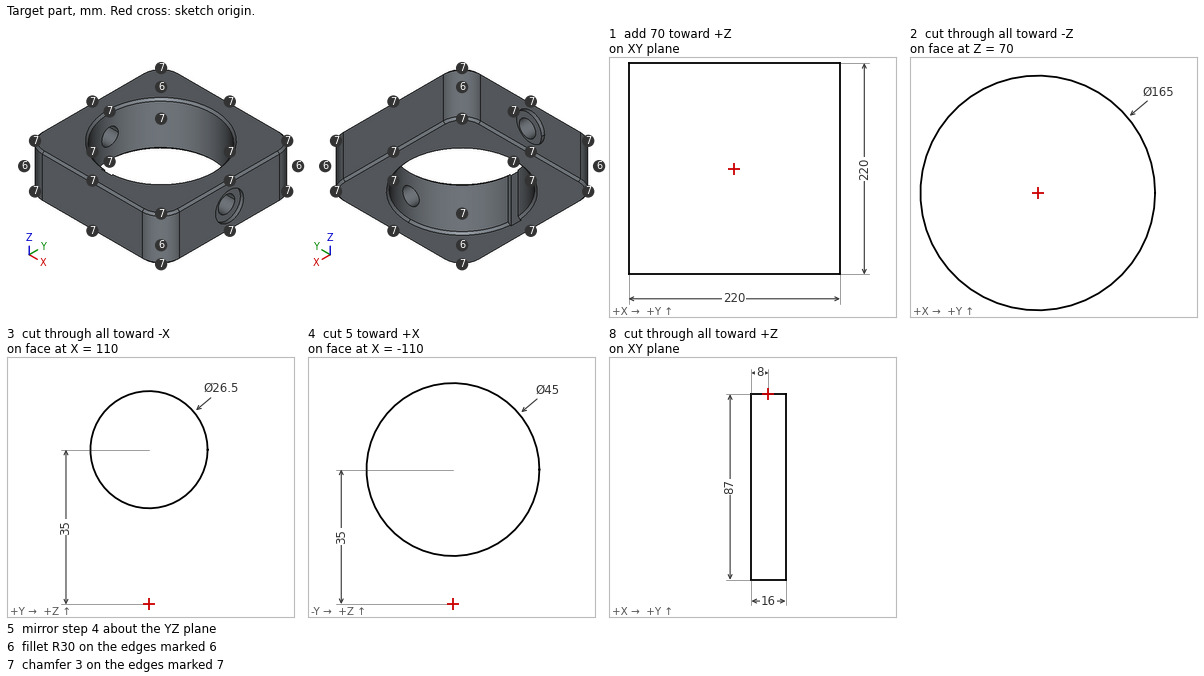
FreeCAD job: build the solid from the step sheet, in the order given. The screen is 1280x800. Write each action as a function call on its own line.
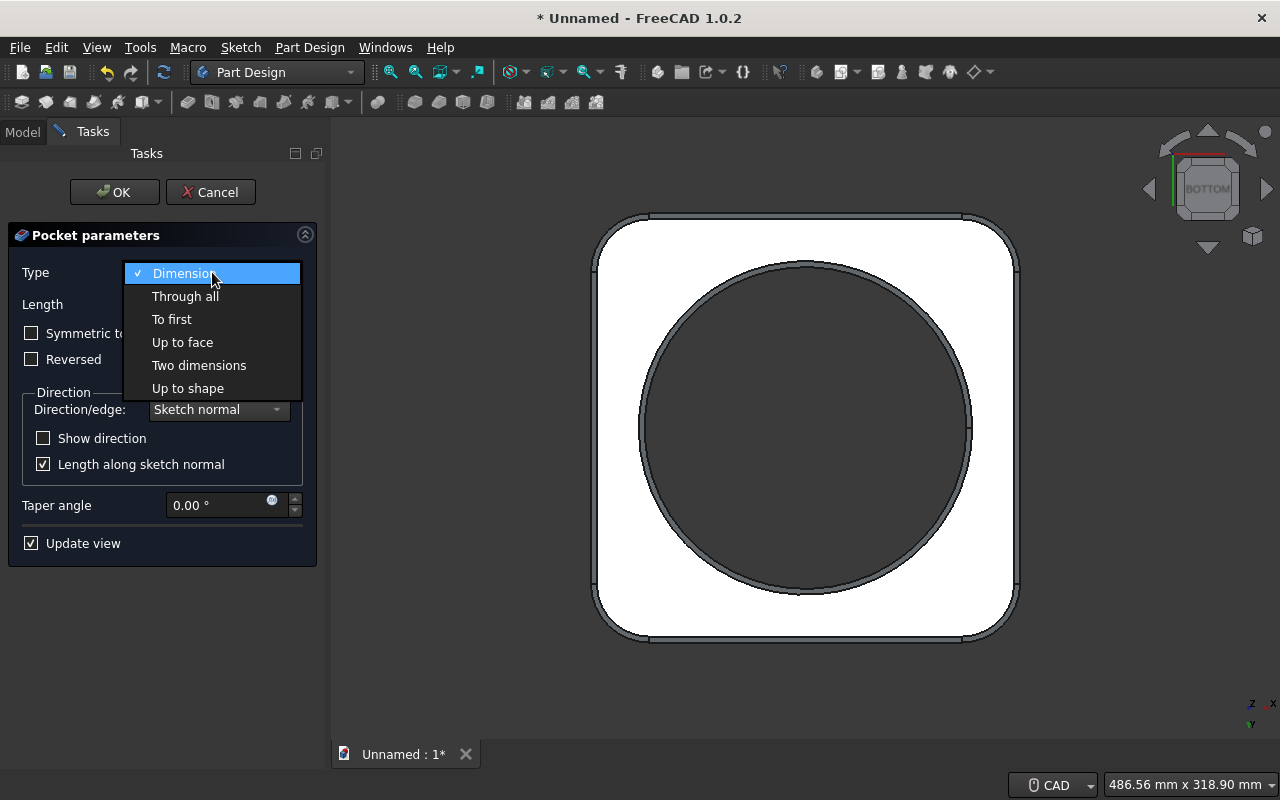
click(212, 296)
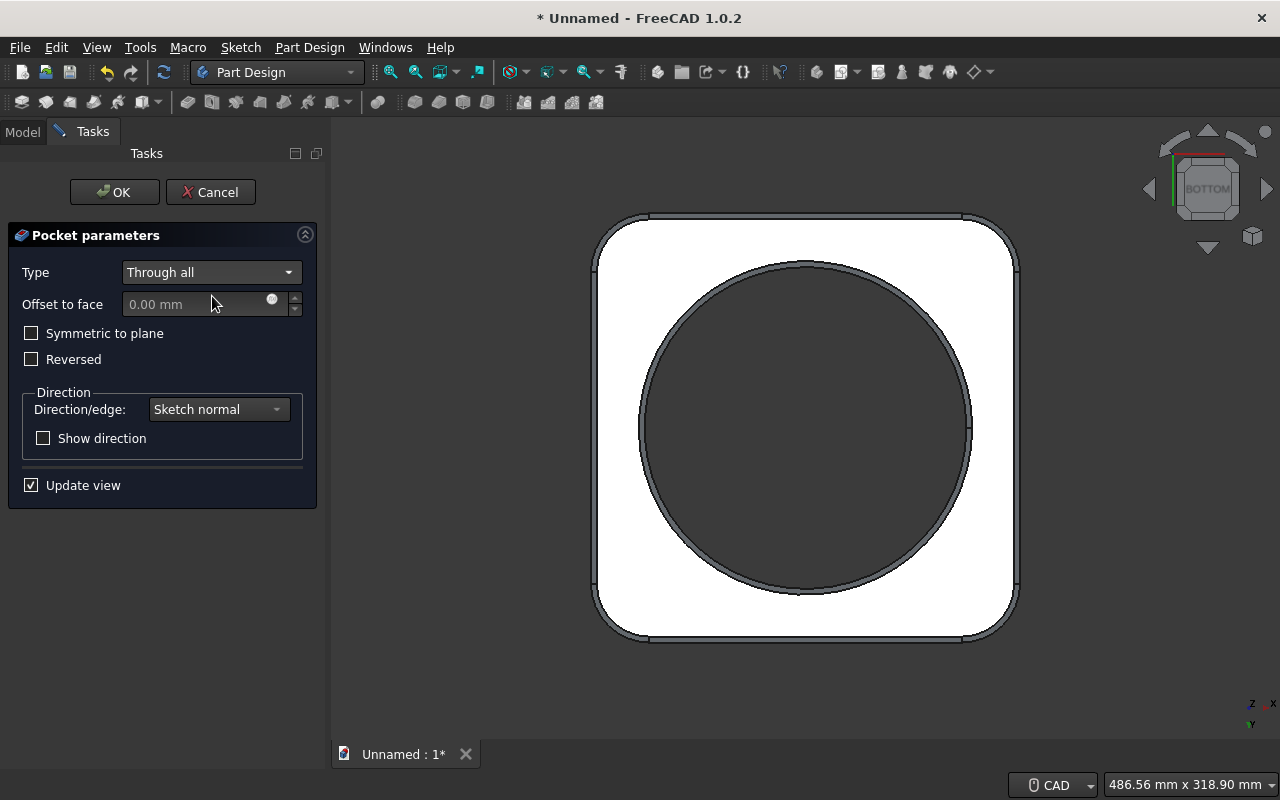
click(30, 359)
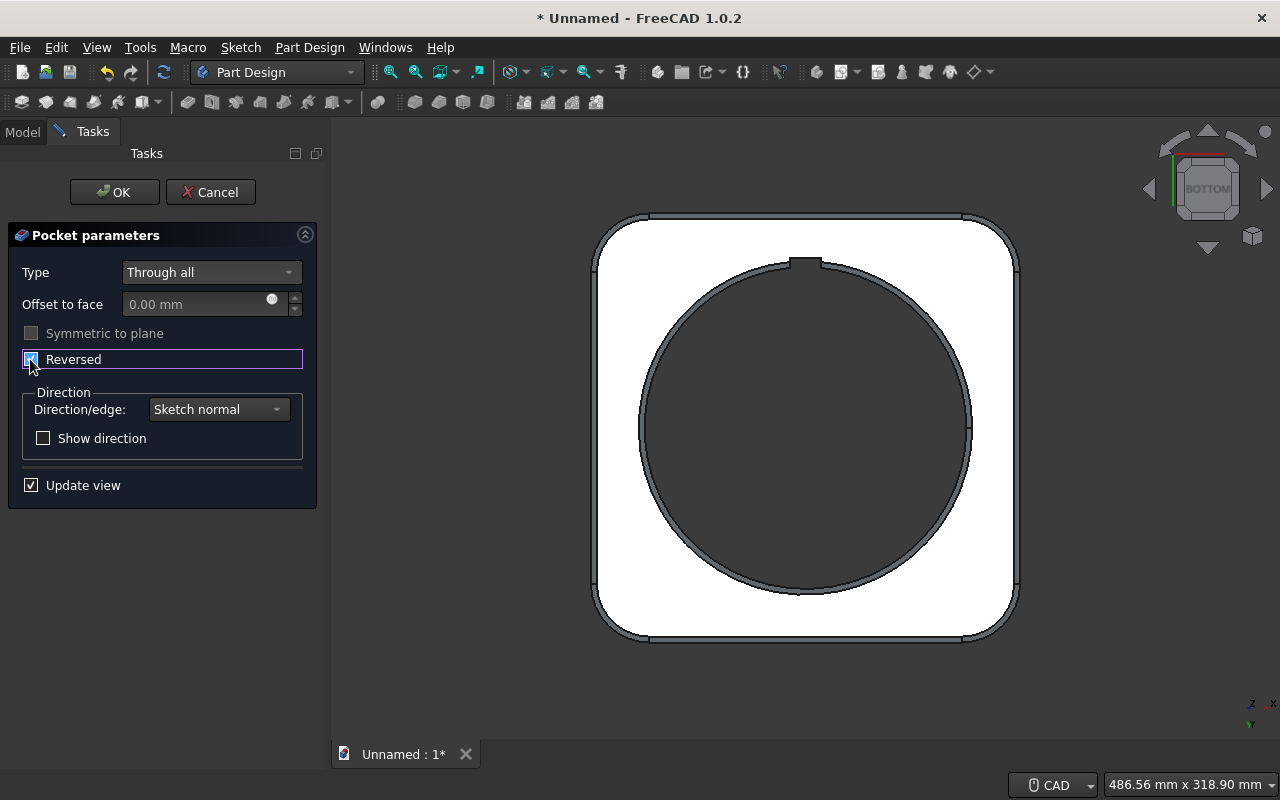
click(115, 192)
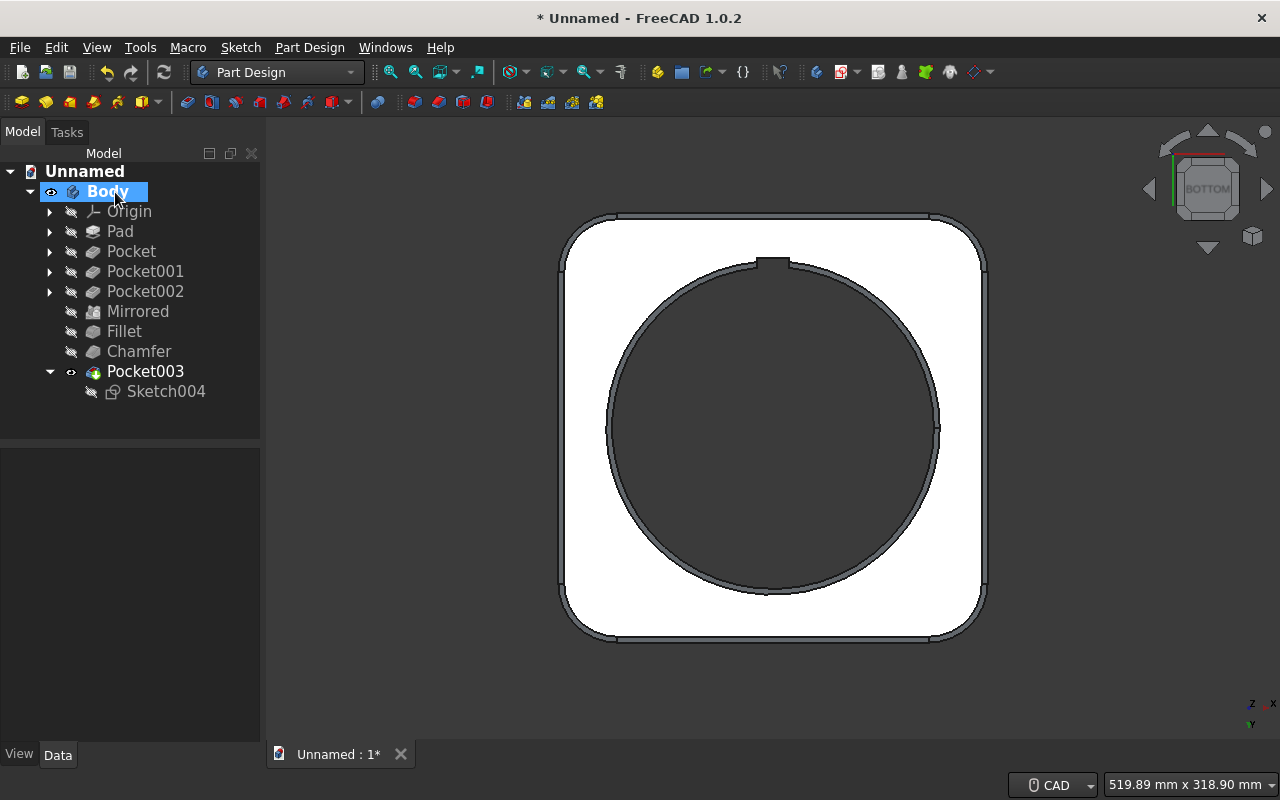
key(0)